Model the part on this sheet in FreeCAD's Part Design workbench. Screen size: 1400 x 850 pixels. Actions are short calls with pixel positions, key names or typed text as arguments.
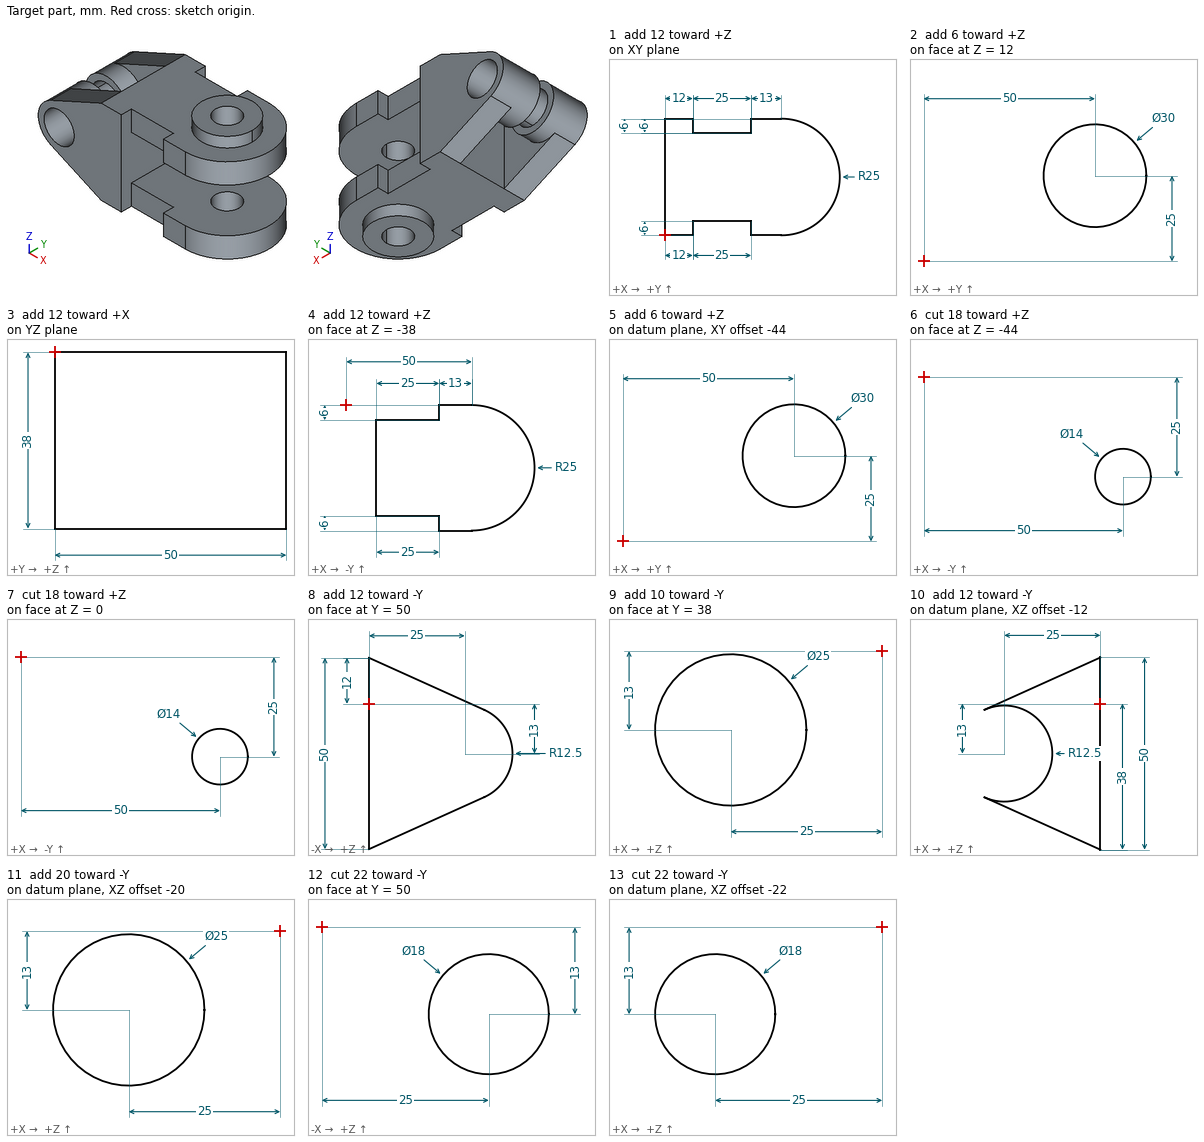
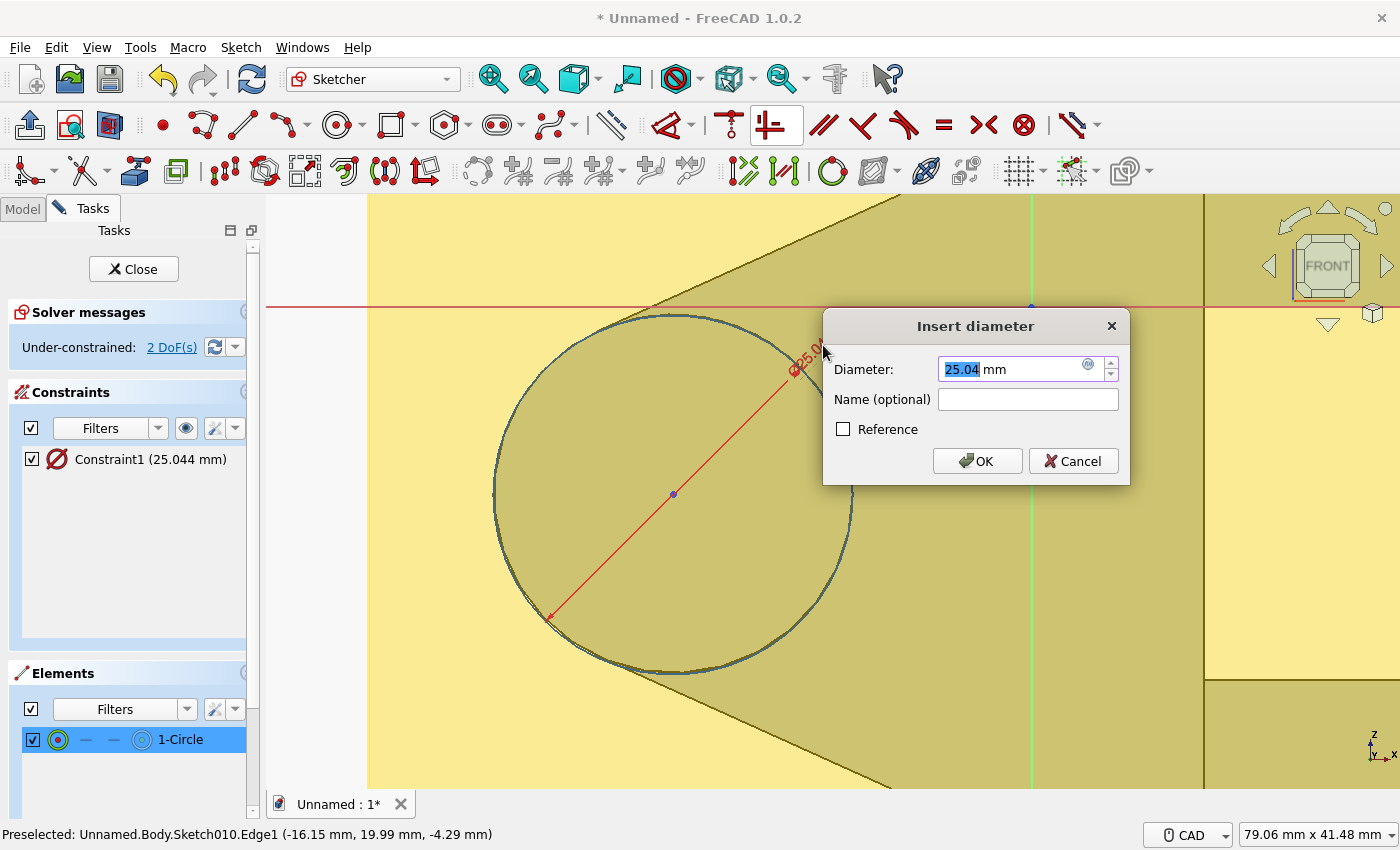
text(25)
key(Return)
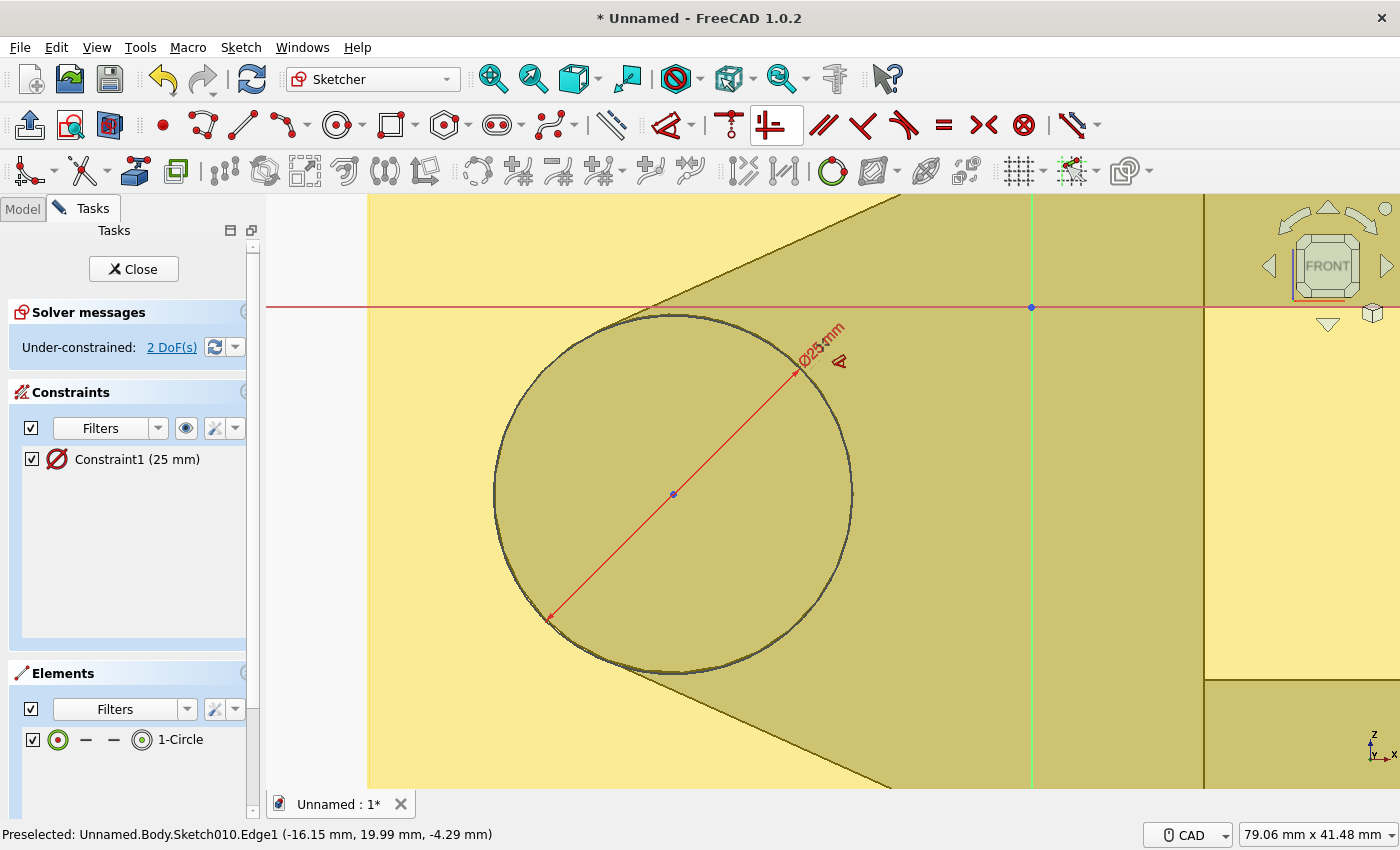
click(673, 495)
click(852, 273)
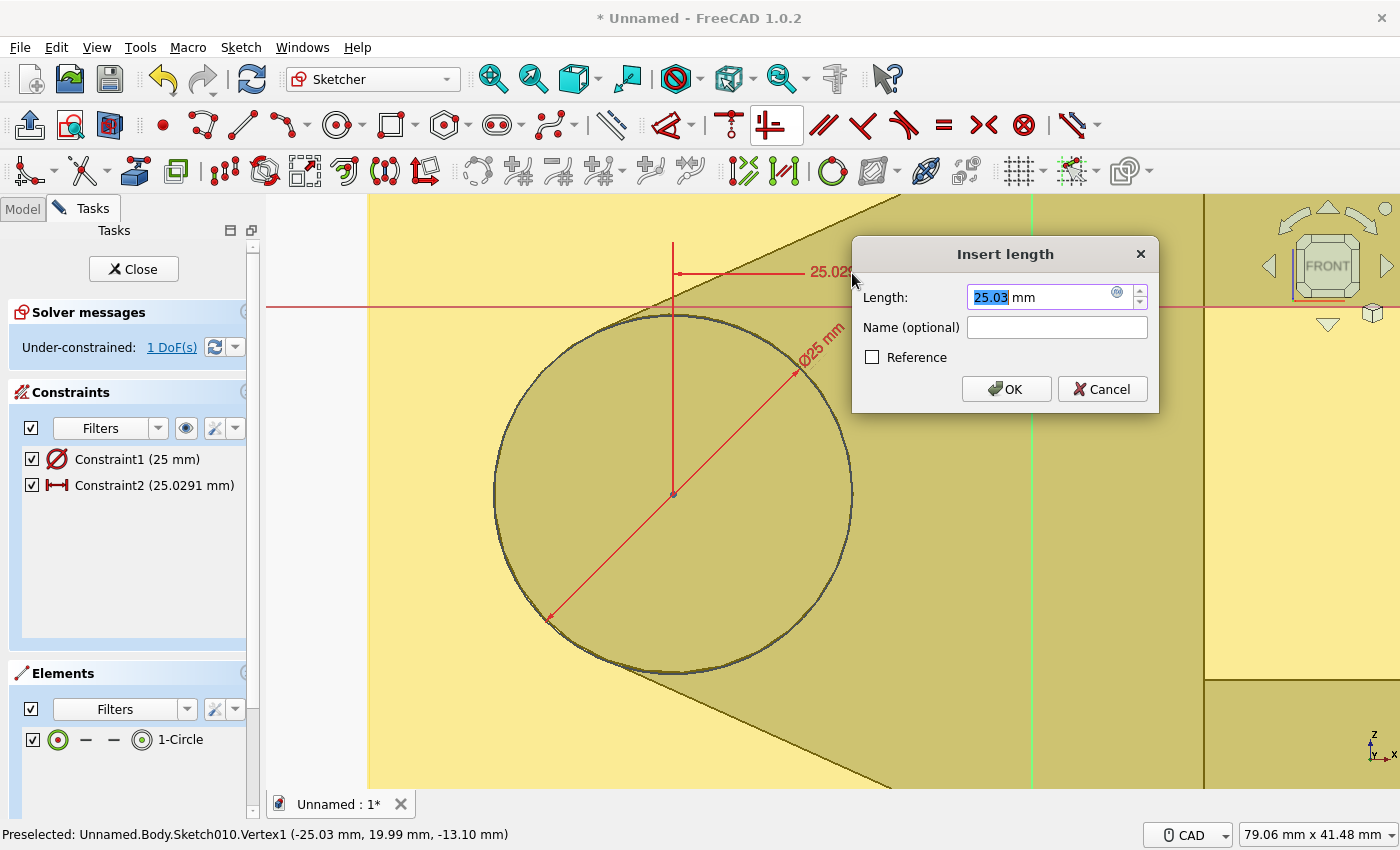
text(25)
key(Return)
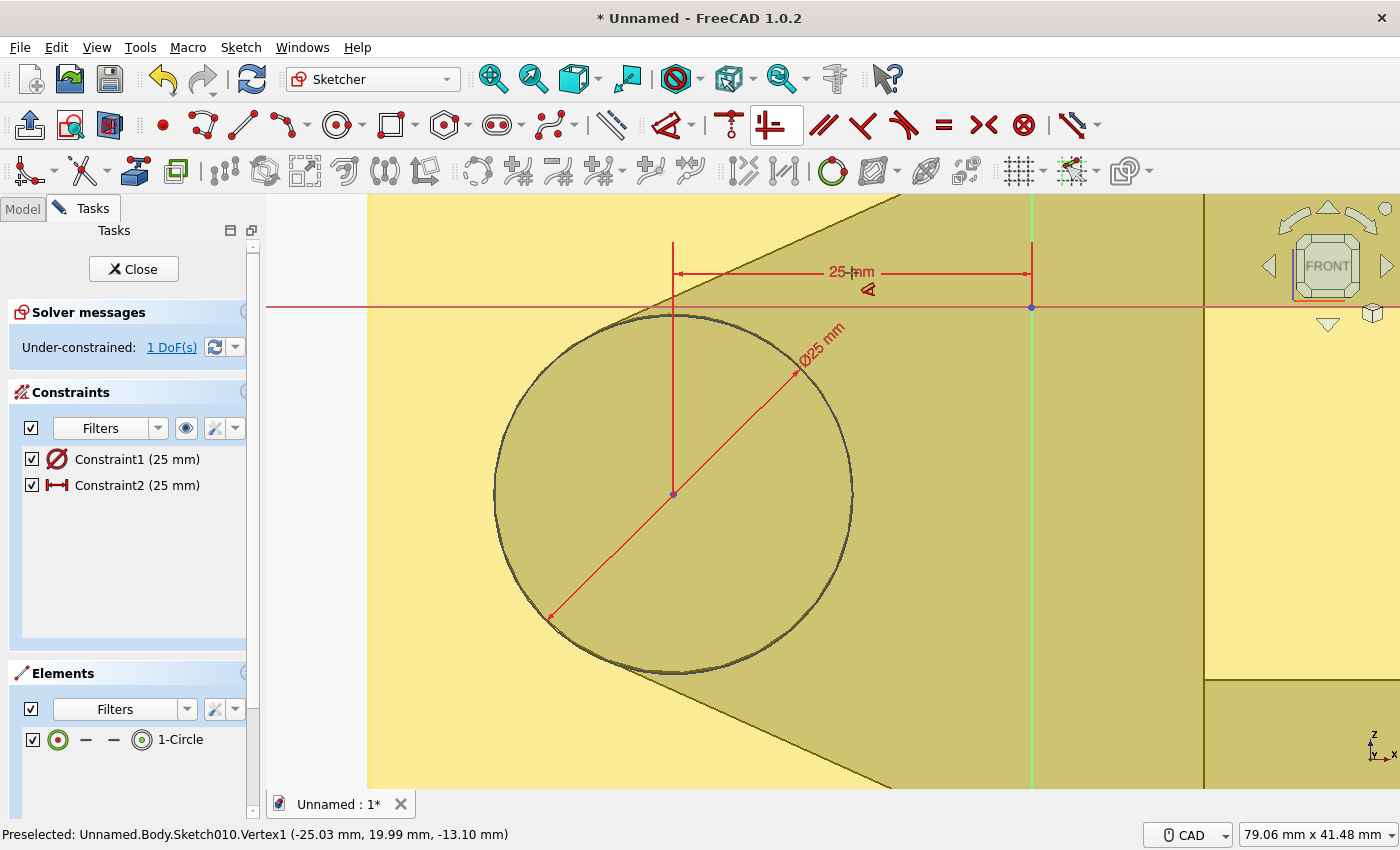
click(673, 495)
click(1066, 401)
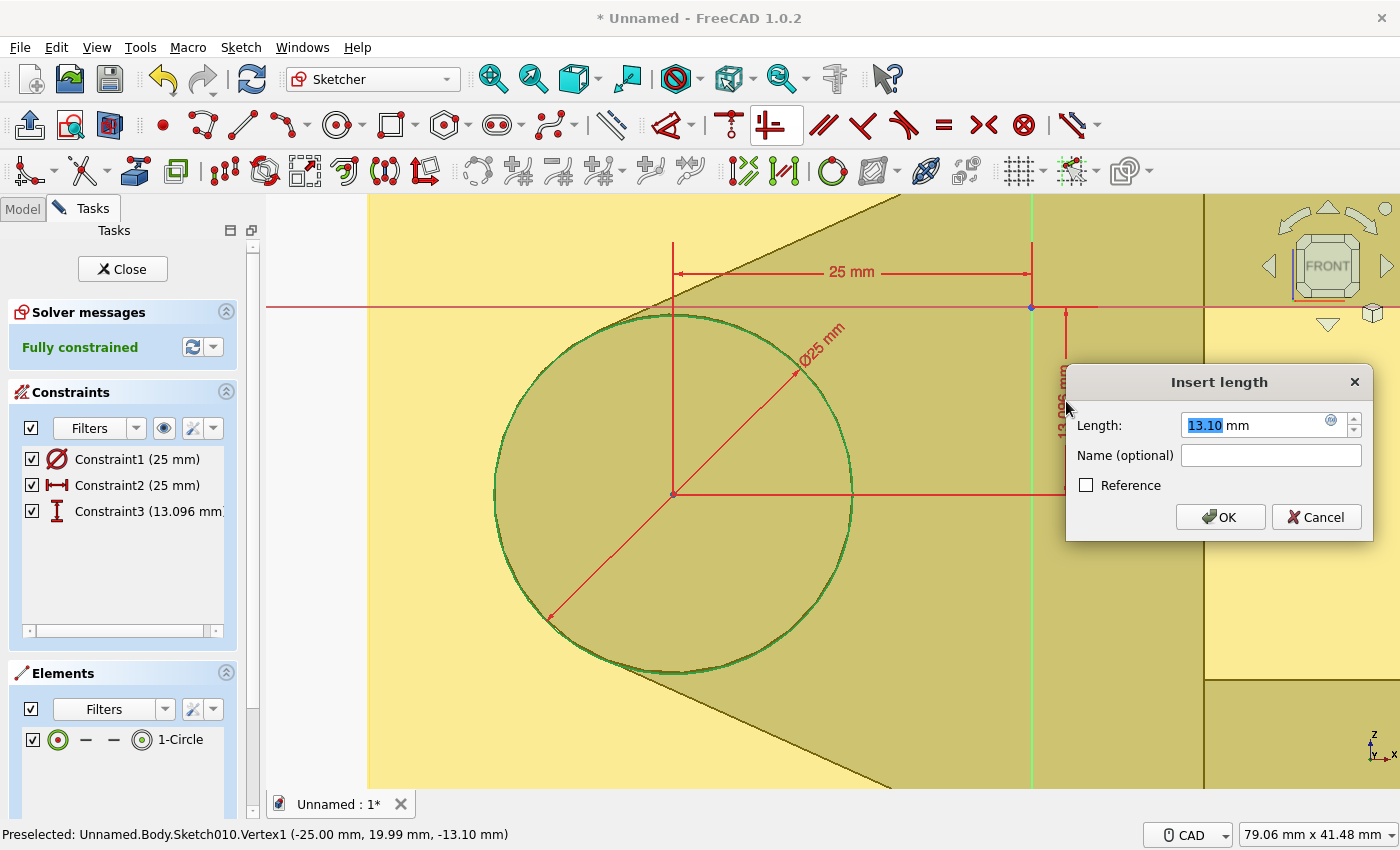
text(13)
key(Return)
key(Escape)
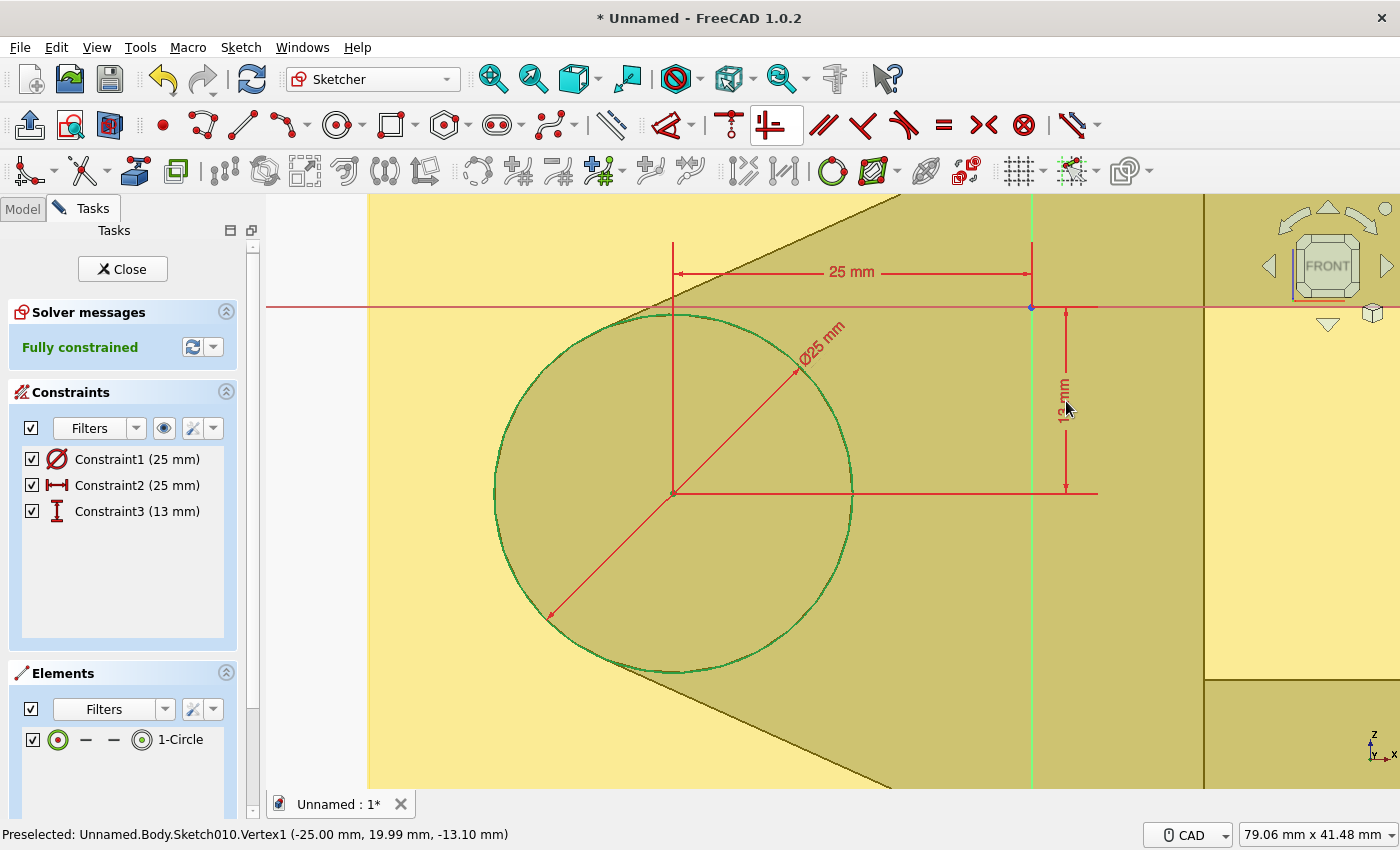
click(123, 269)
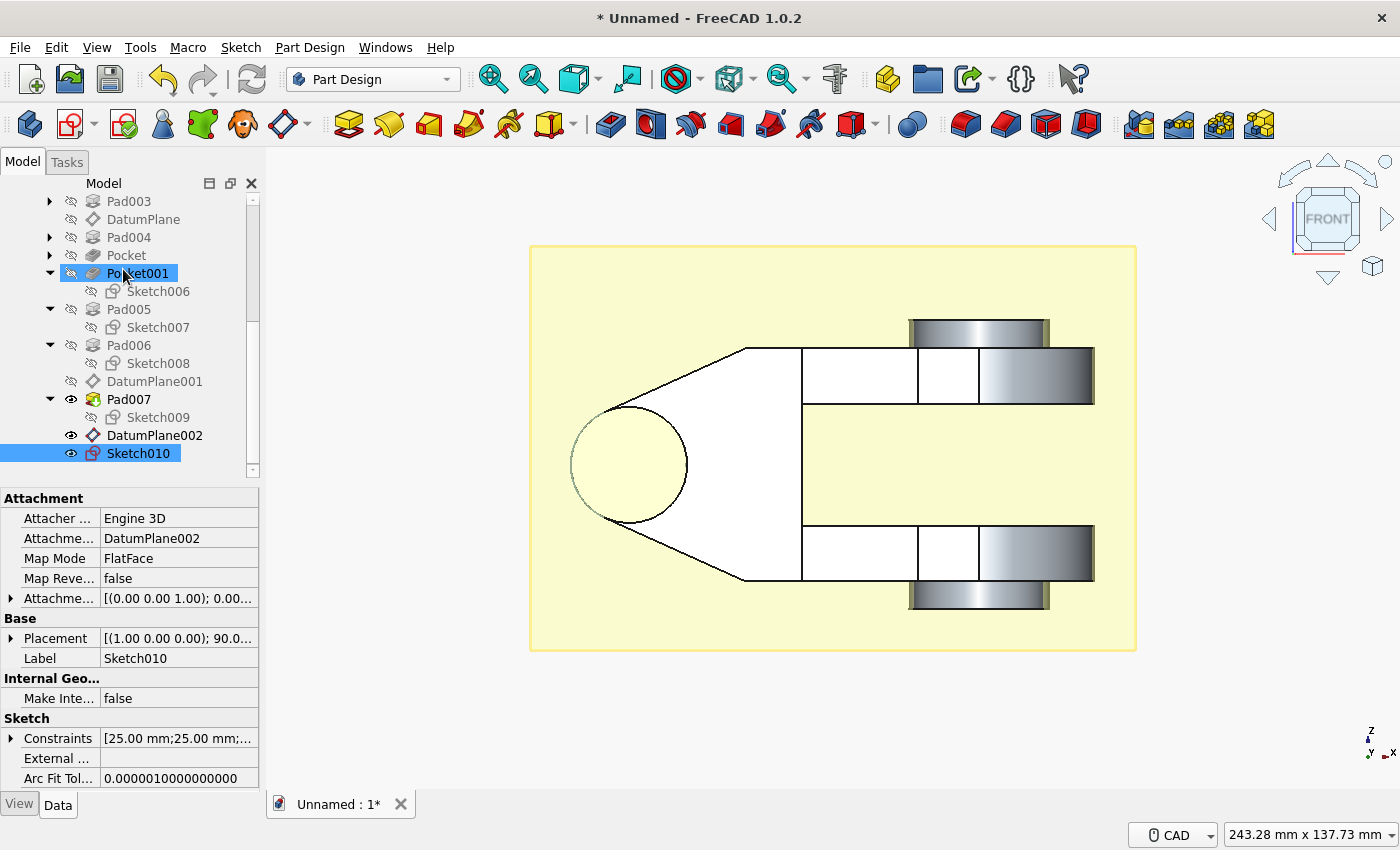
click(350, 124)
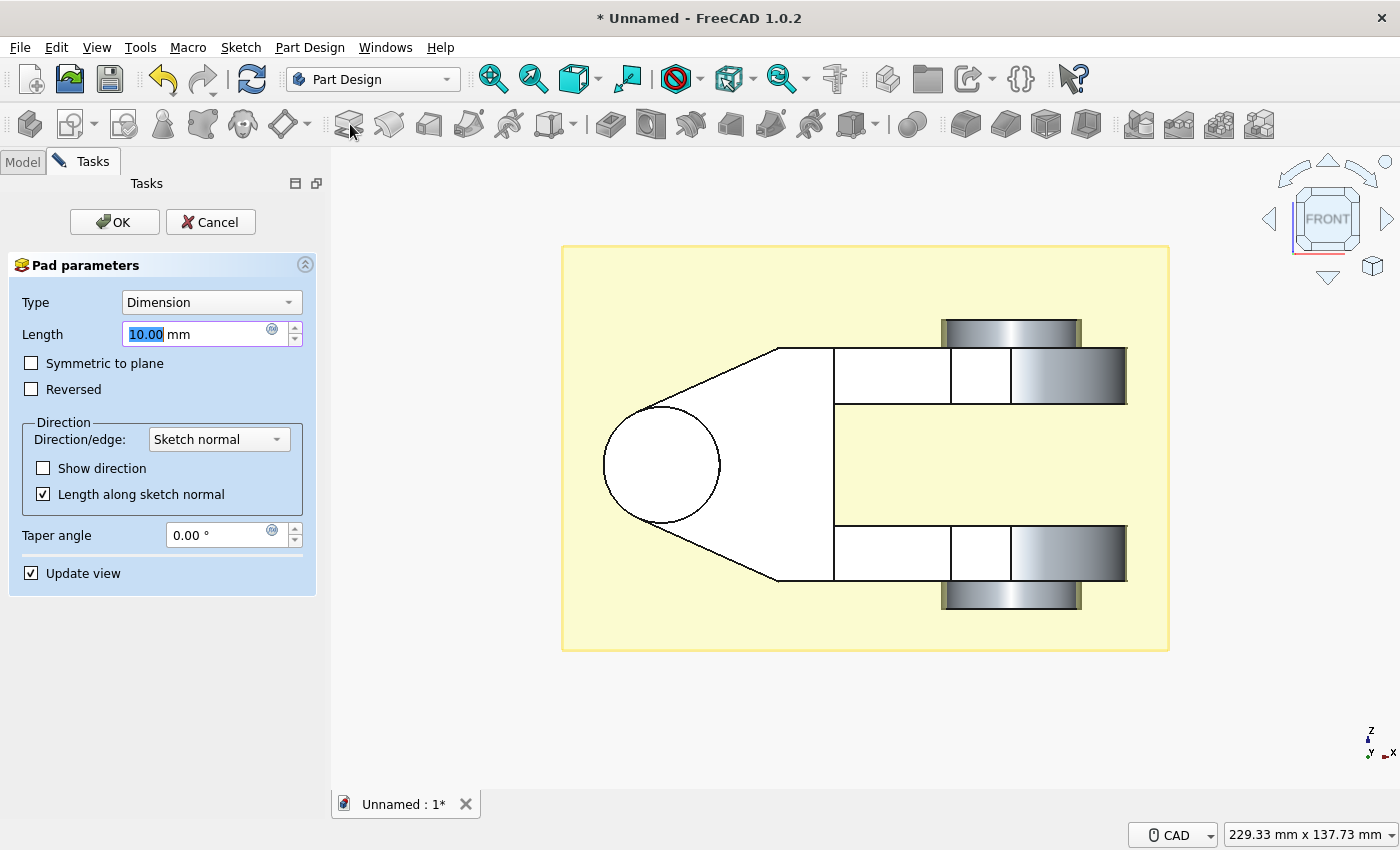
text(20)
key(Tab)